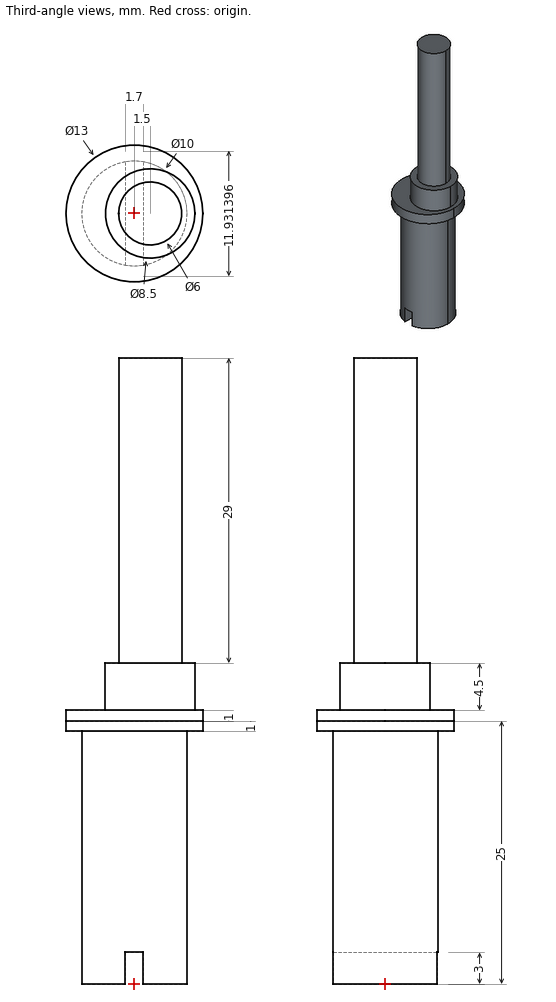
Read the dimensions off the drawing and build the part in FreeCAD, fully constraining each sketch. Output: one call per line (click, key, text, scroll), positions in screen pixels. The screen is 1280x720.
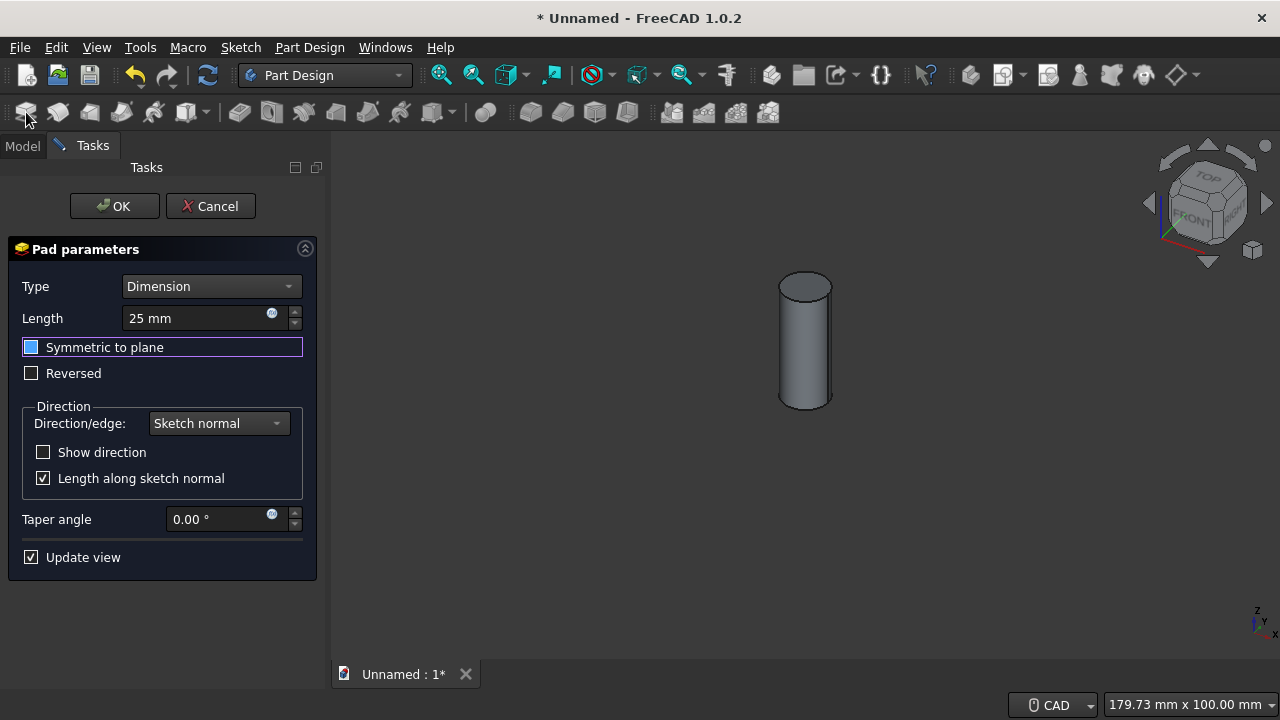
click(115, 206)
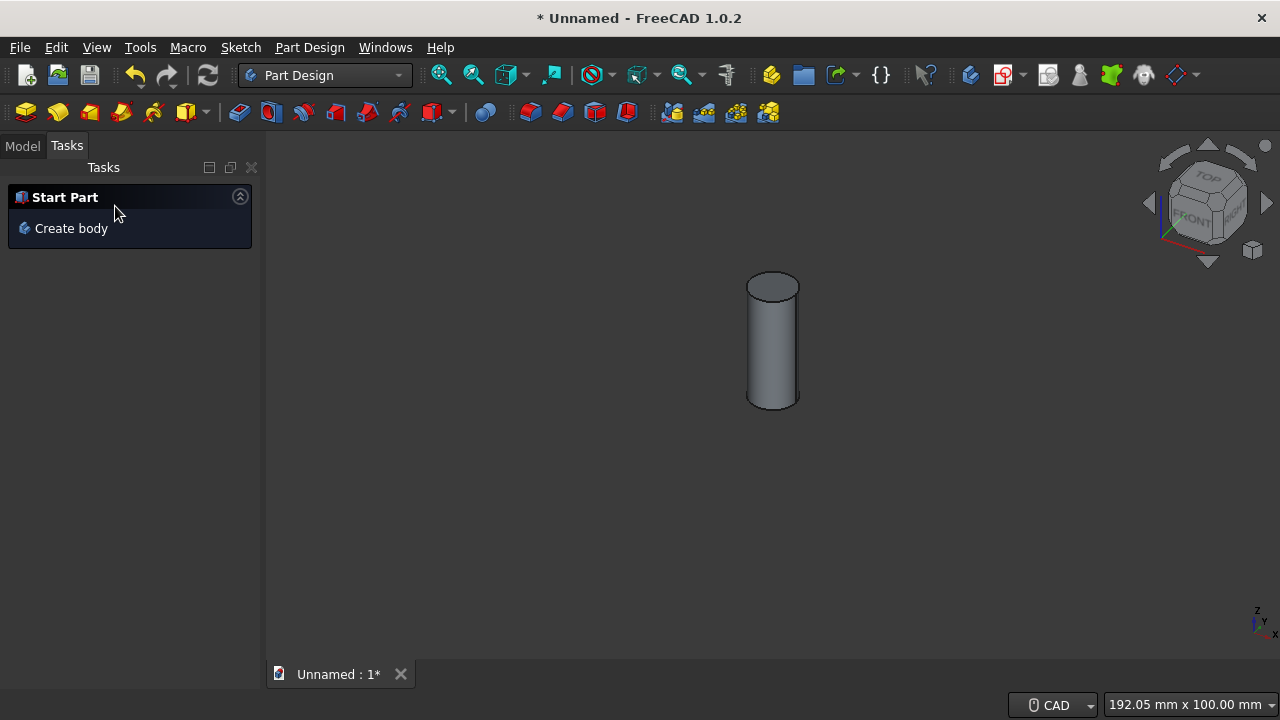
click(442, 76)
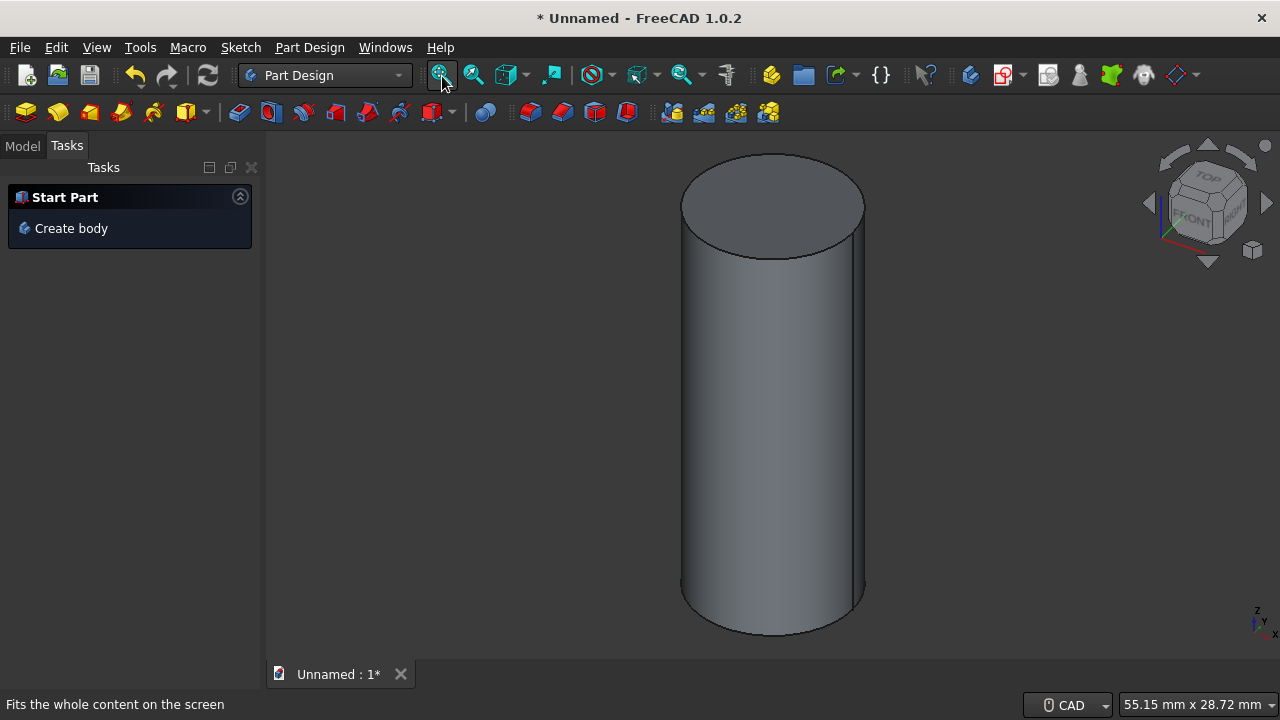
click(773, 206)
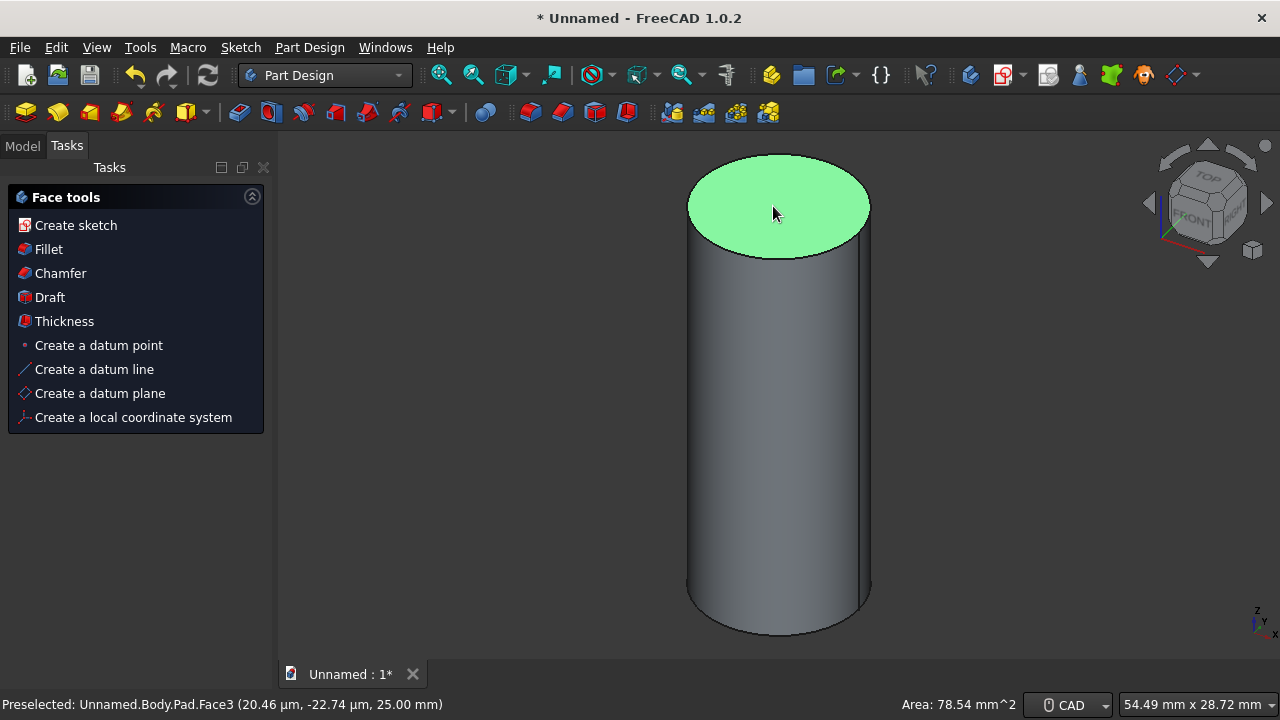
click(1004, 76)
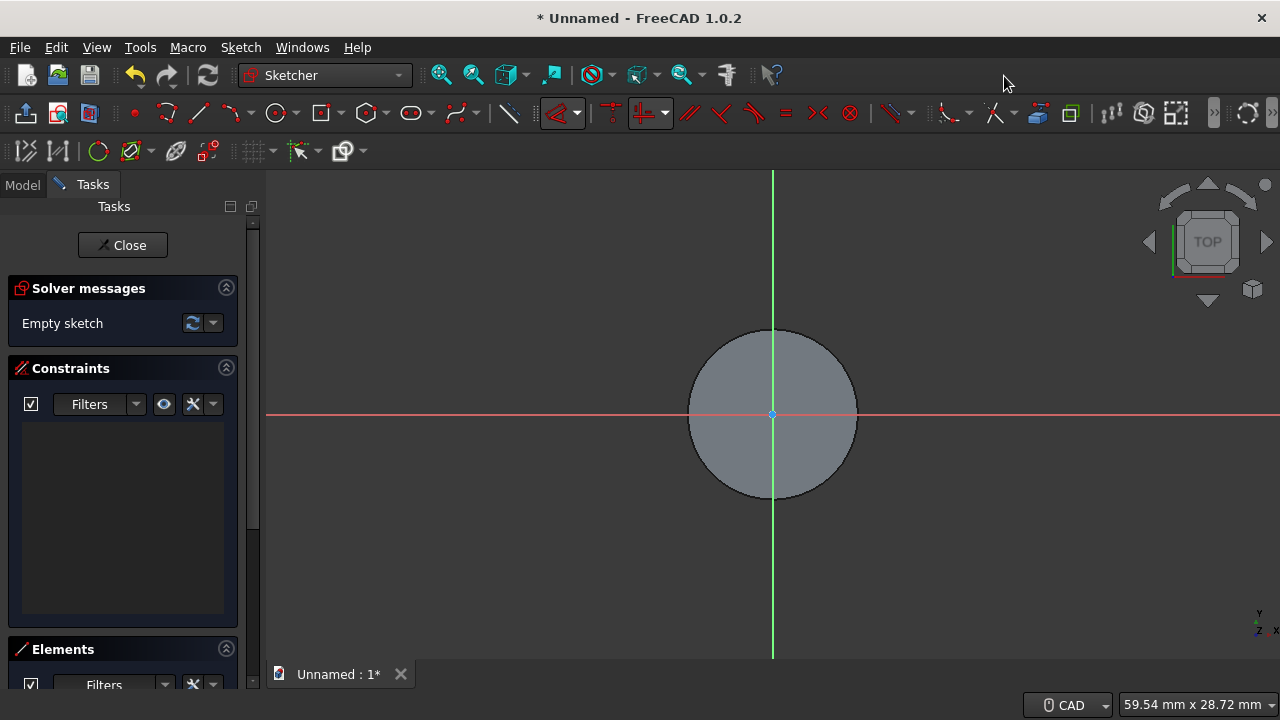
scroll(912, 414, up, 2)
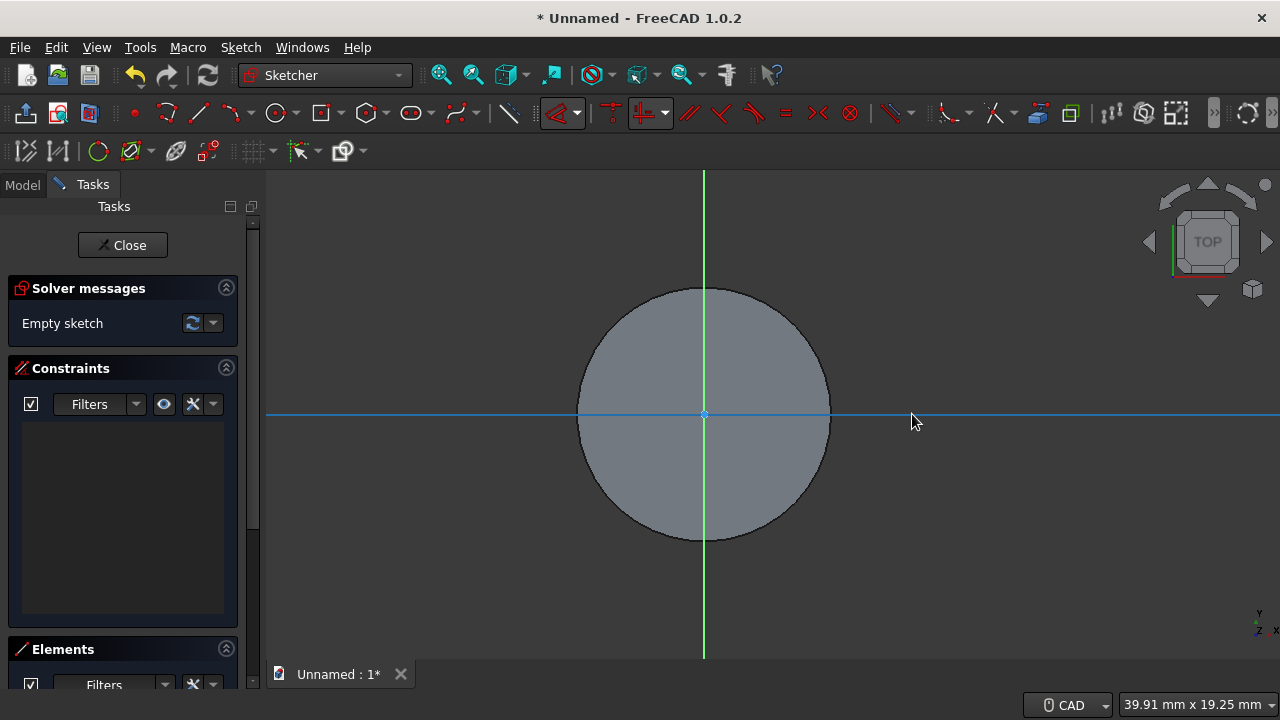
click(276, 114)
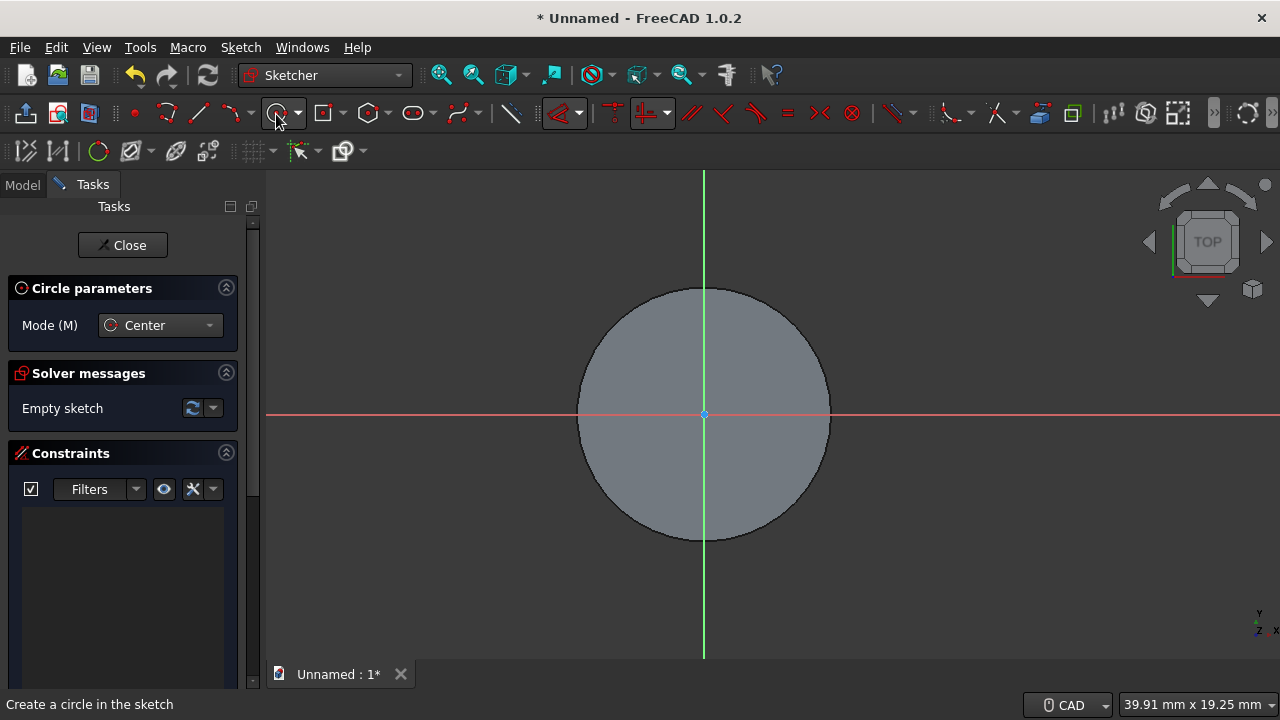
click(704, 414)
move(821, 298)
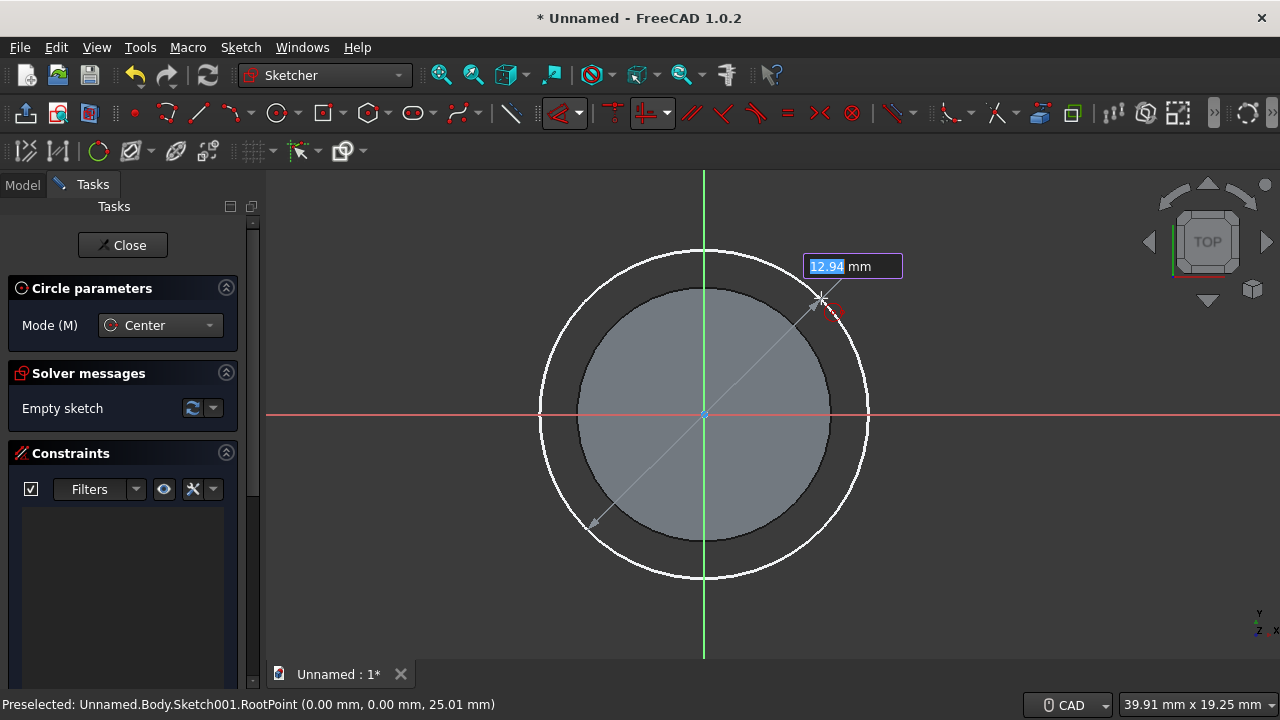
text(13)
key(Return)
key(Escape)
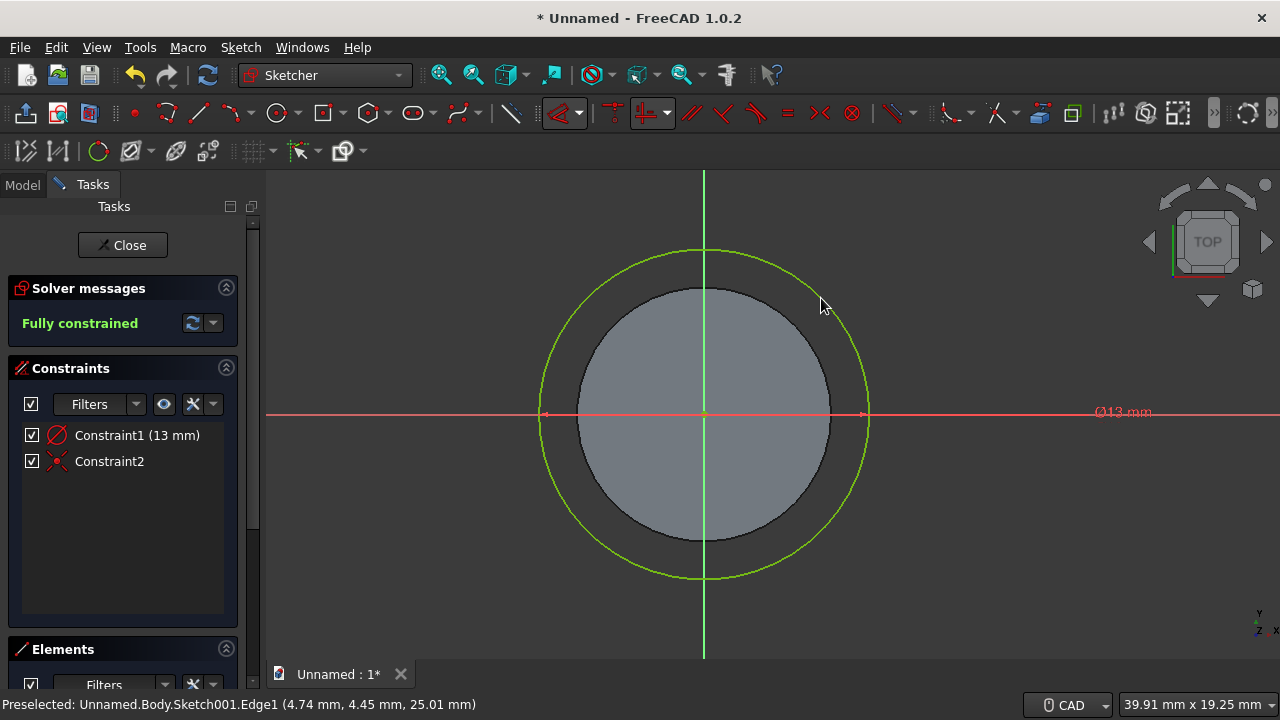
click(123, 245)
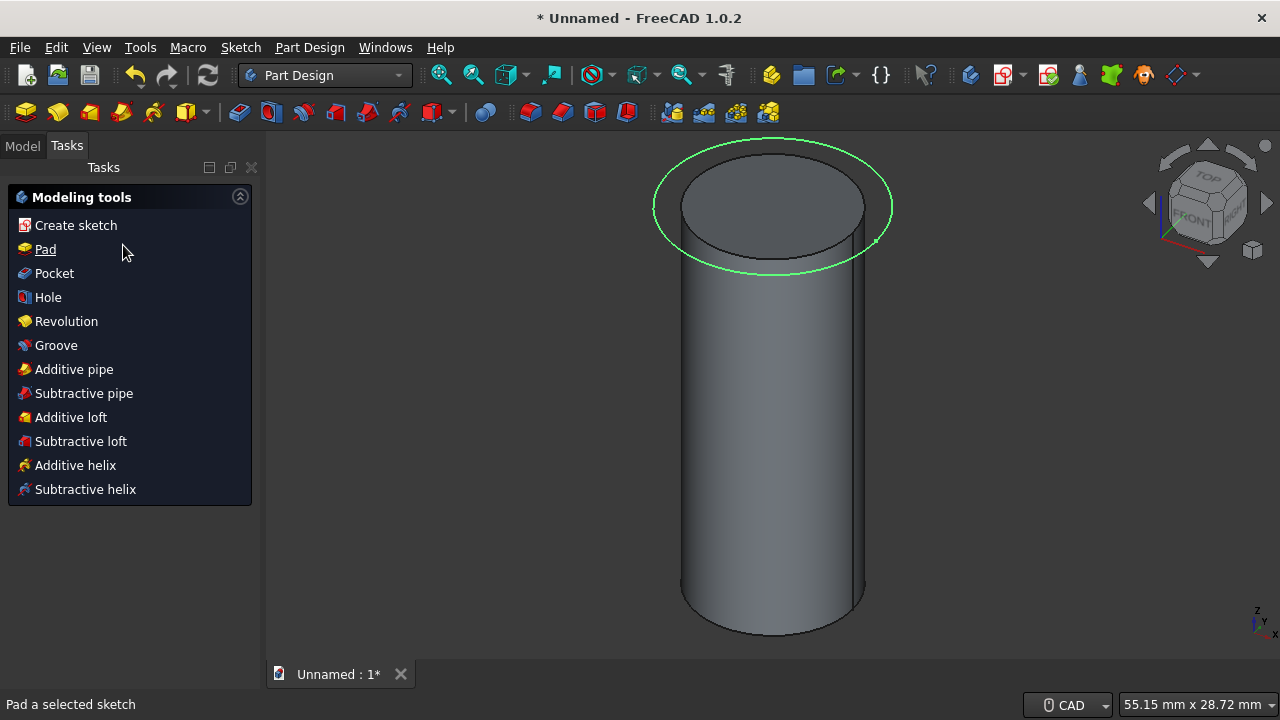
click(26, 112)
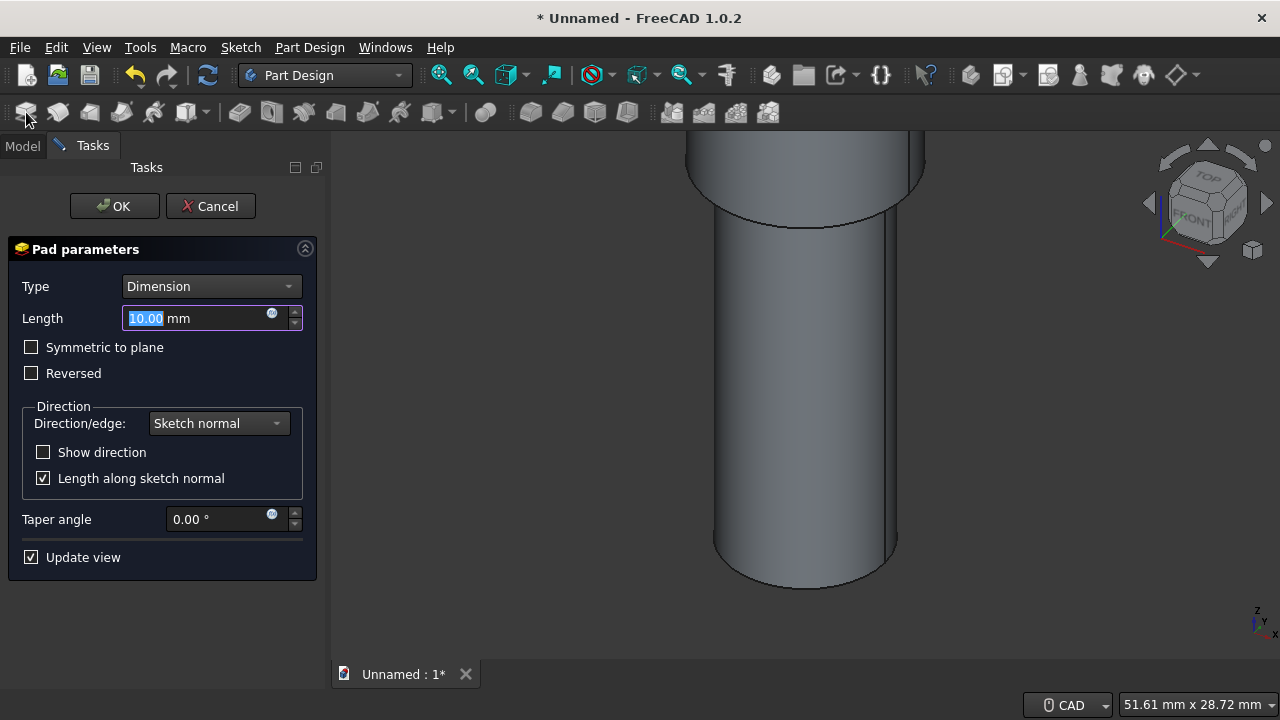
text(1)
key(Tab)